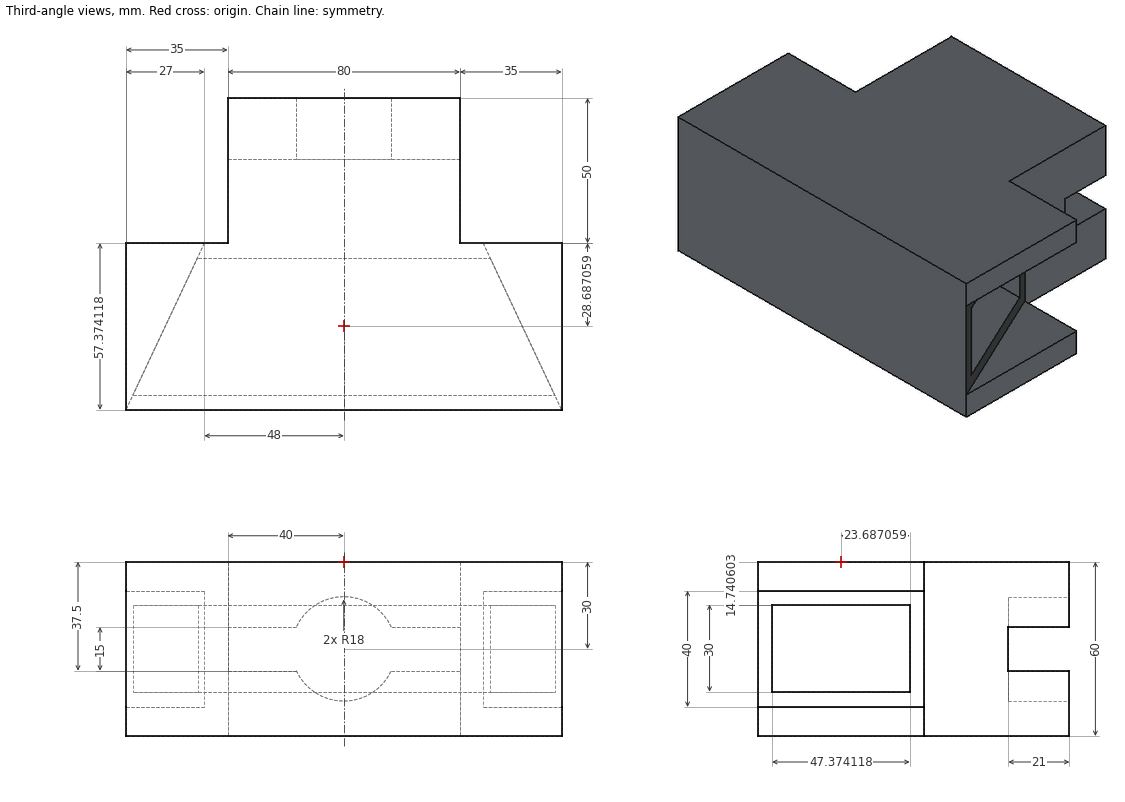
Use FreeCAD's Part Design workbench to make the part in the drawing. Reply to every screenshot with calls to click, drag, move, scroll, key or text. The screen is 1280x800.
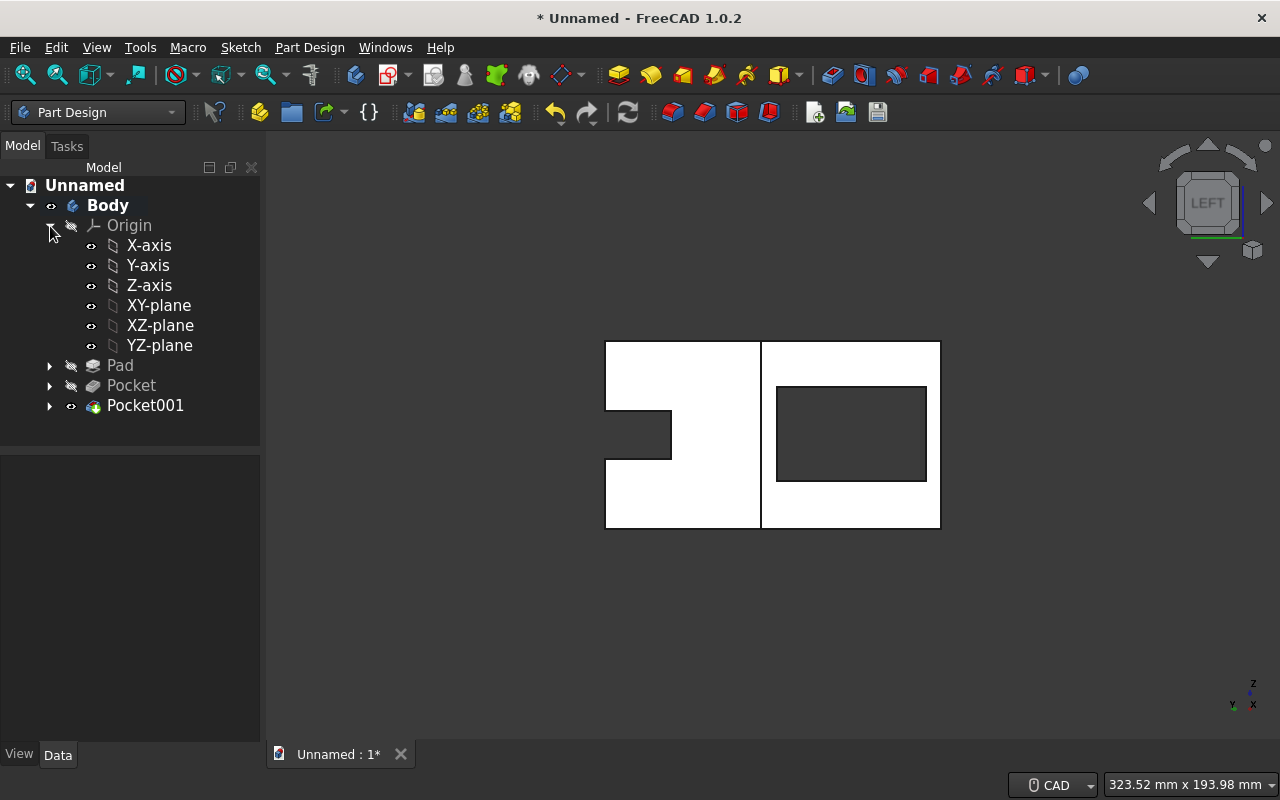
click(136, 306)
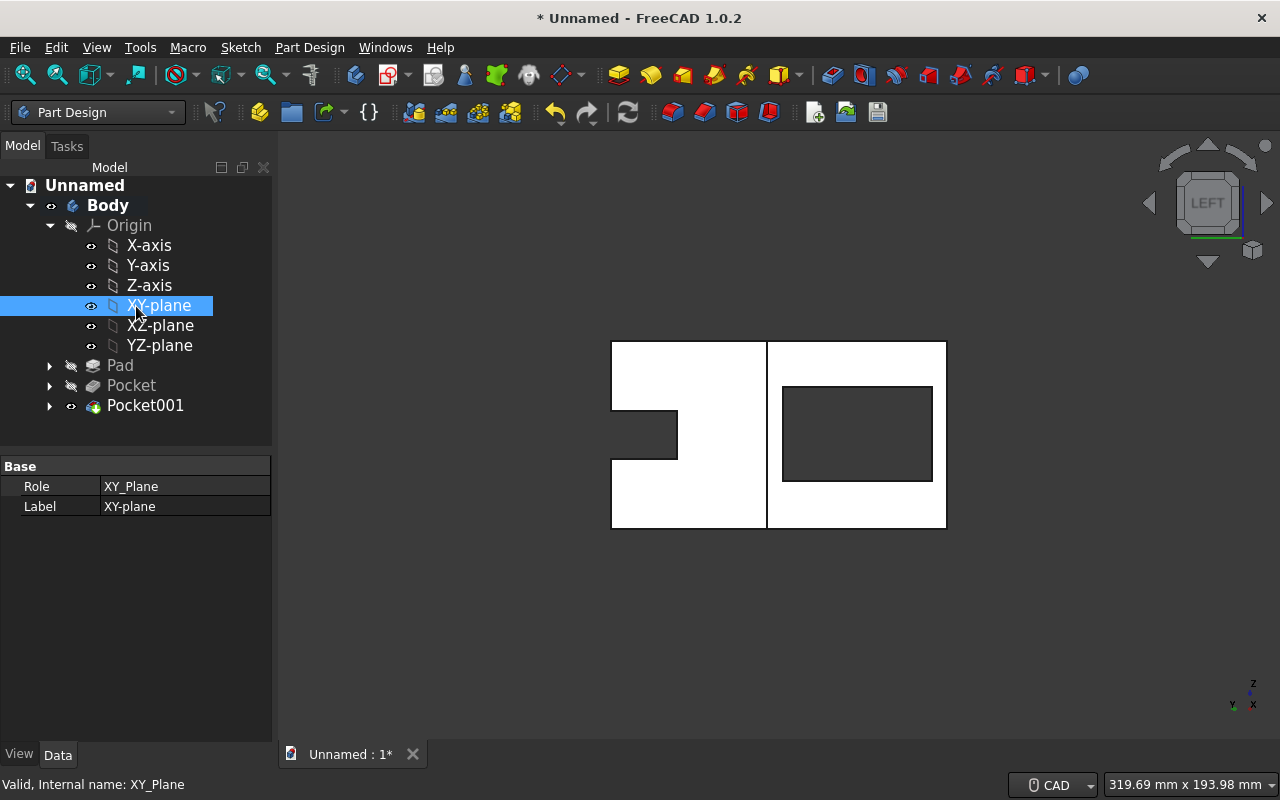
click(562, 76)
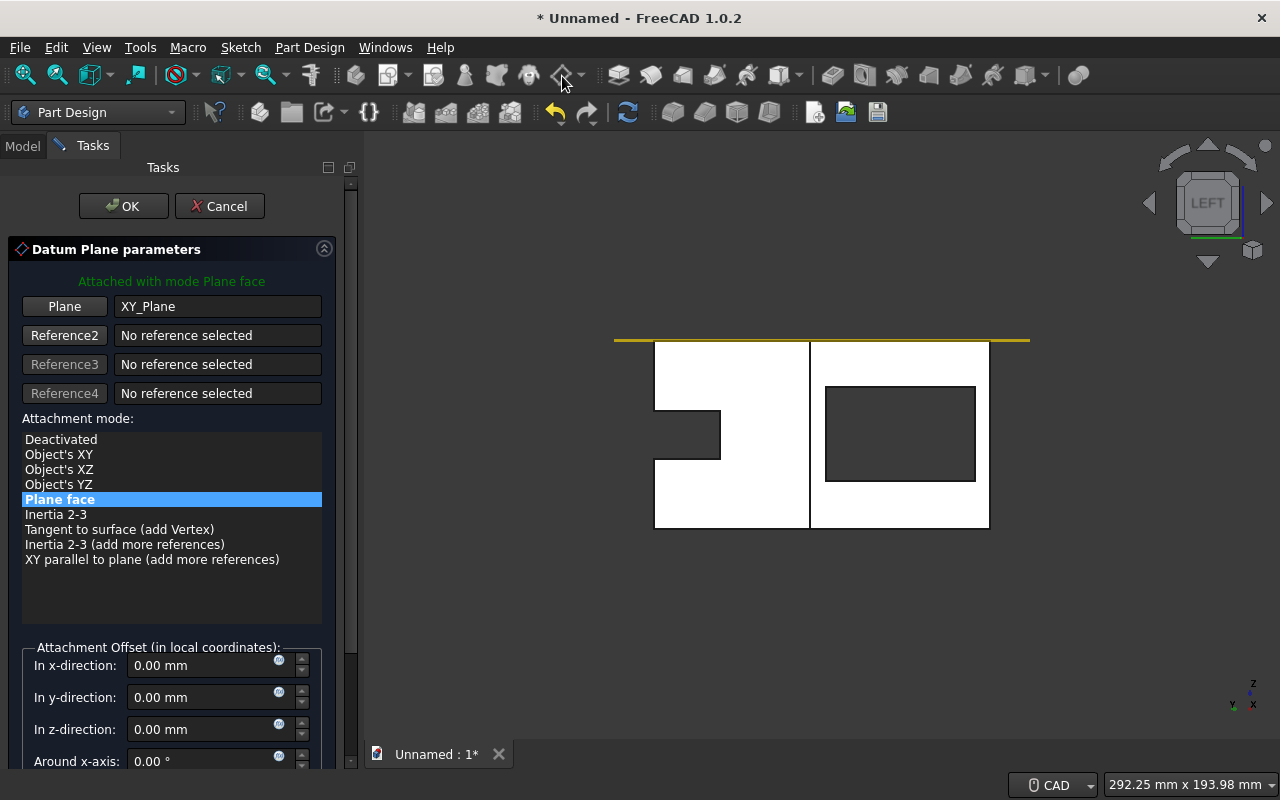
triple_click(210, 729)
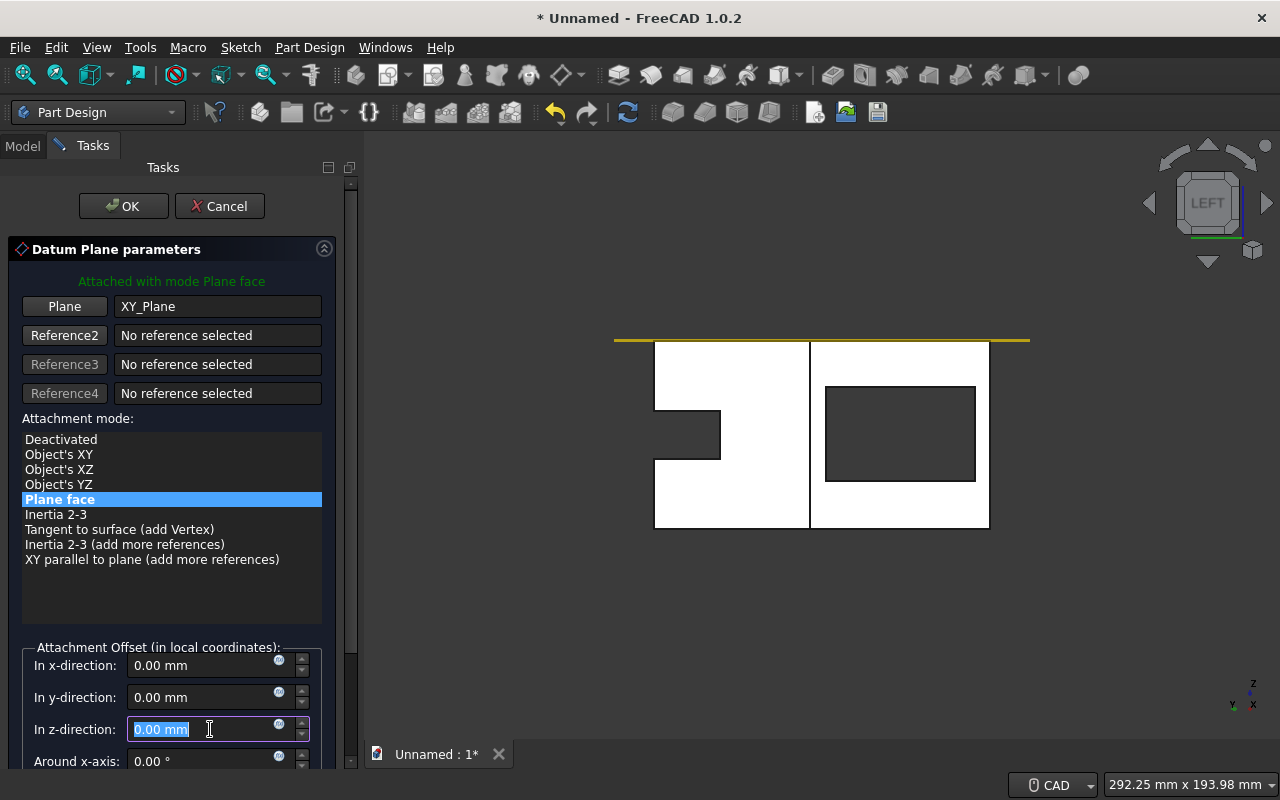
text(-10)
key(Tab)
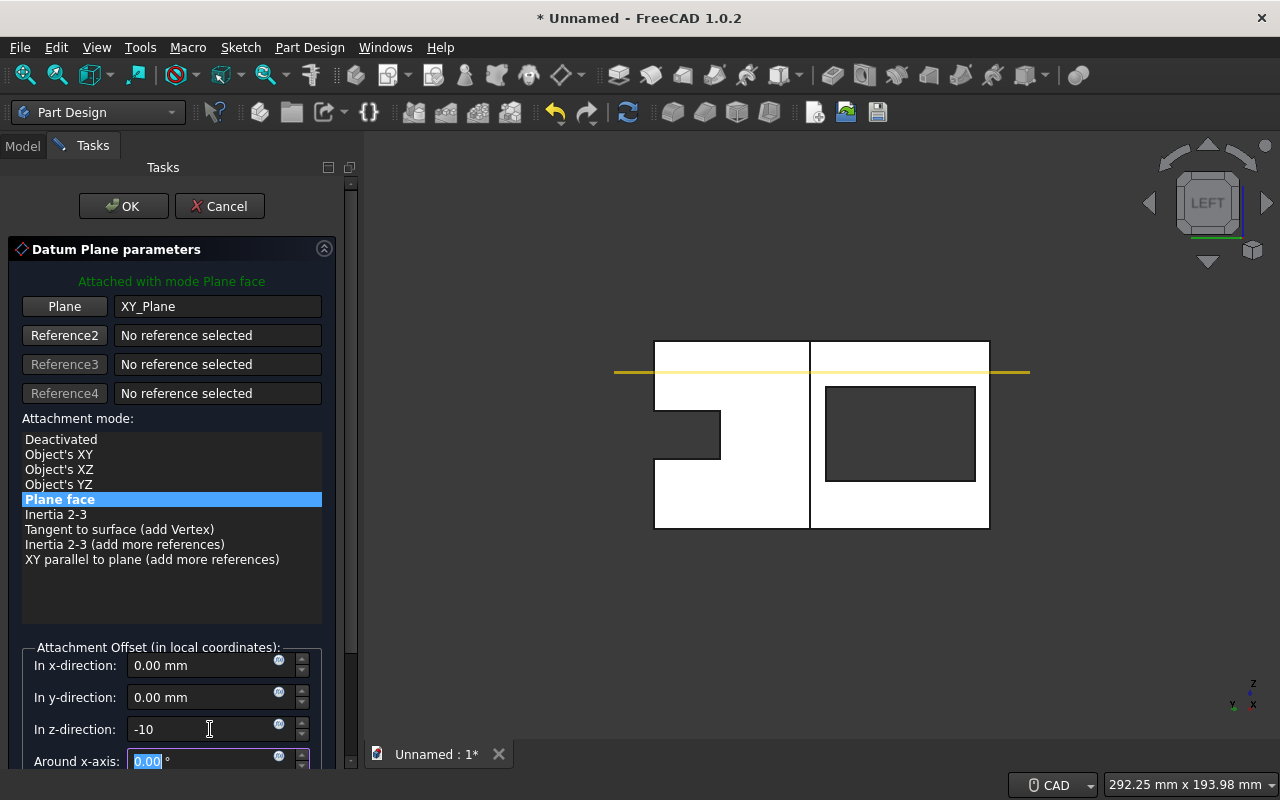
click(124, 206)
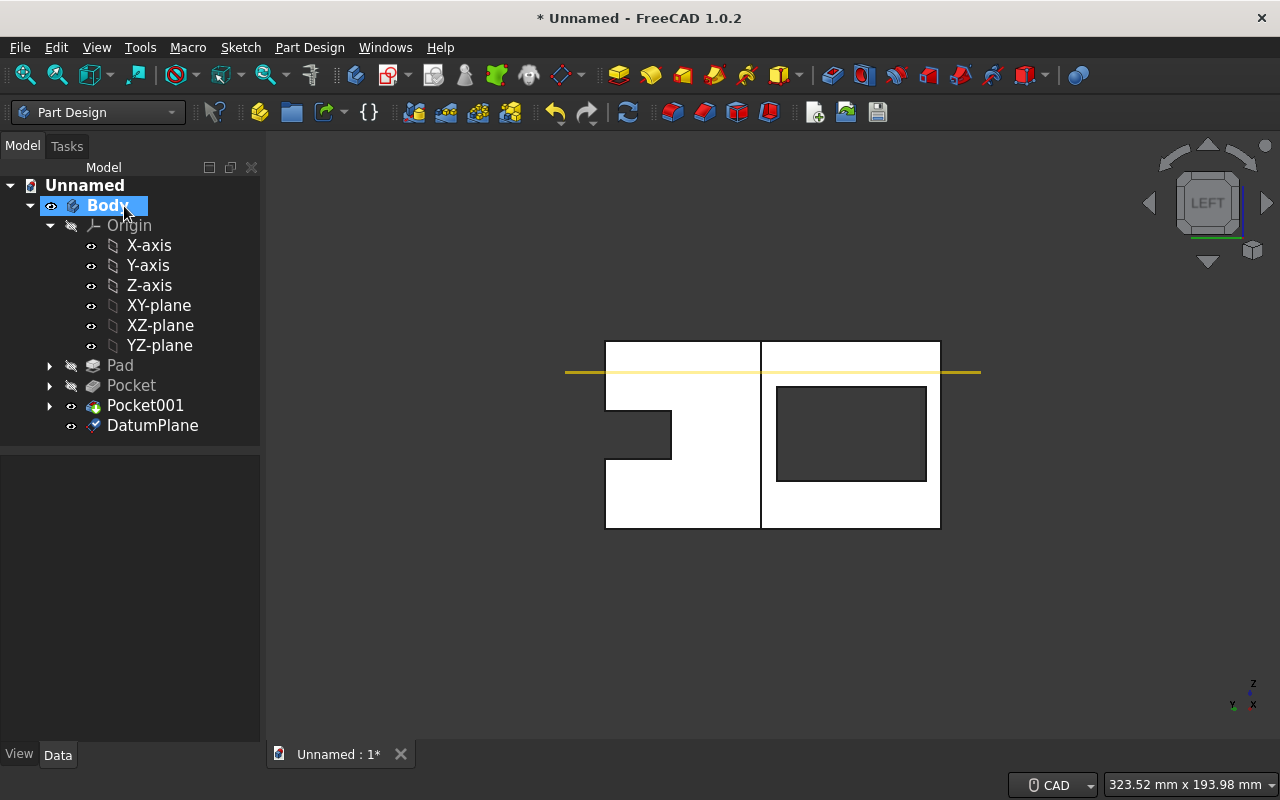
click(116, 426)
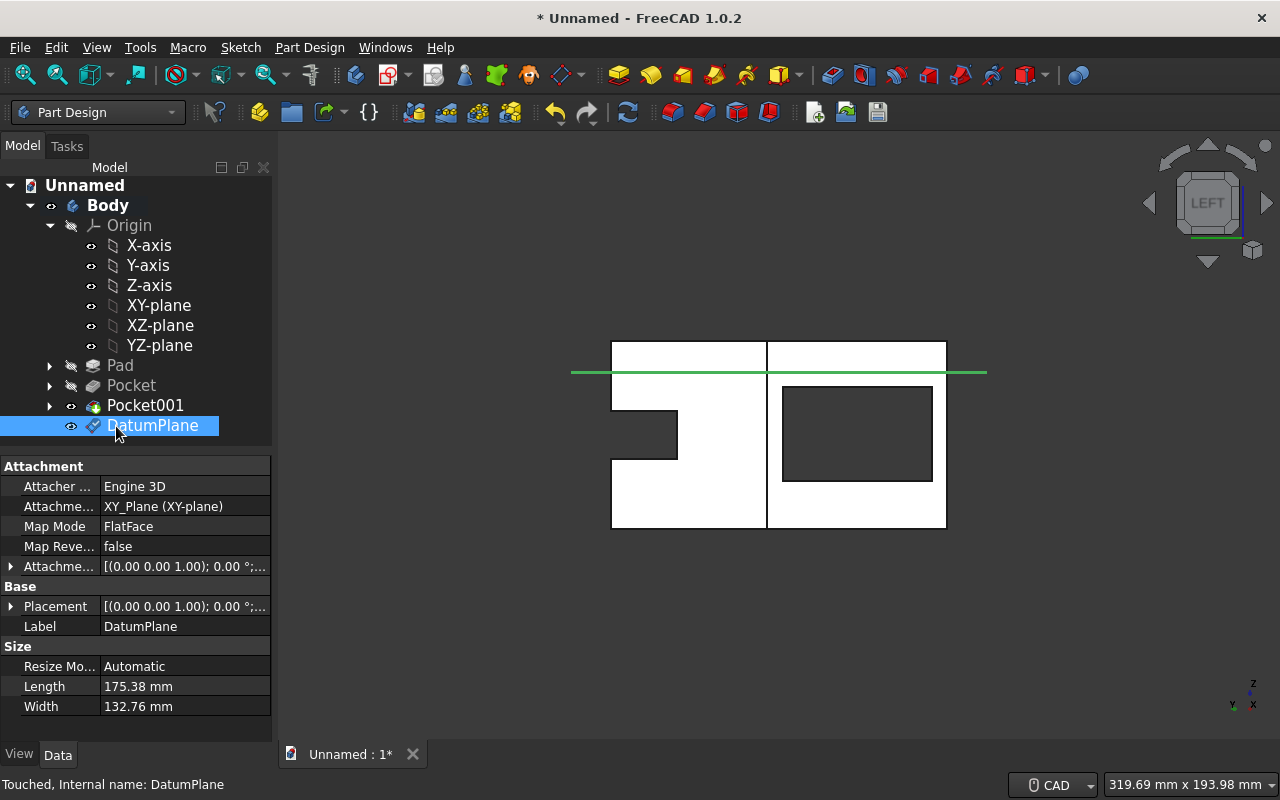
click(388, 76)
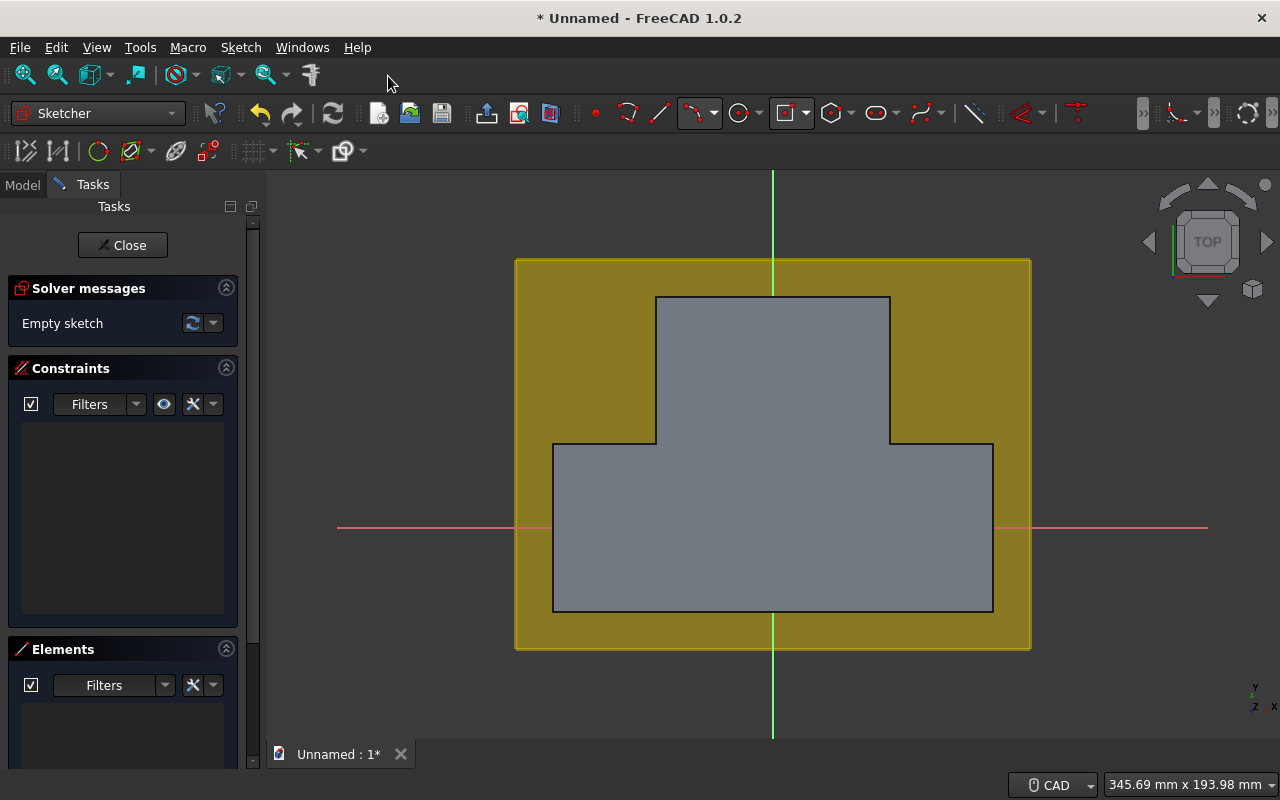
click(552, 114)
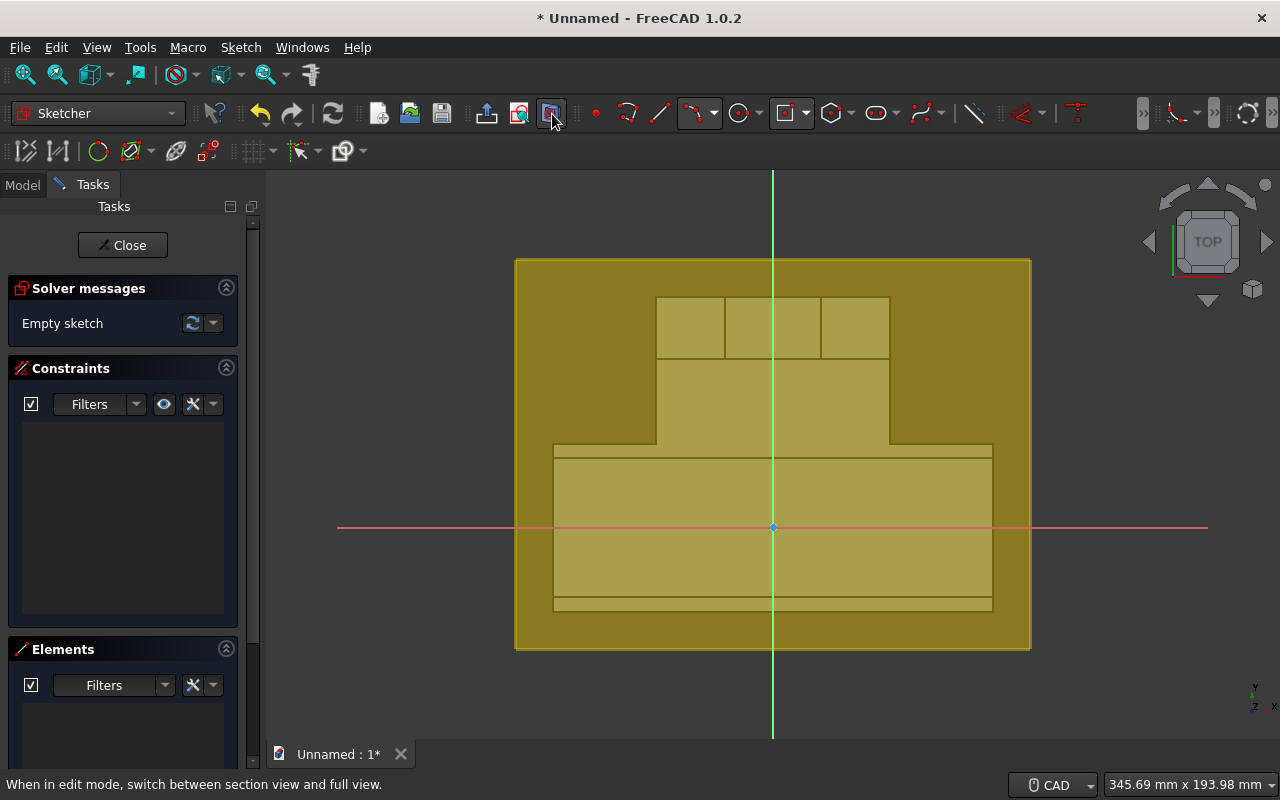
key(g)
key(m)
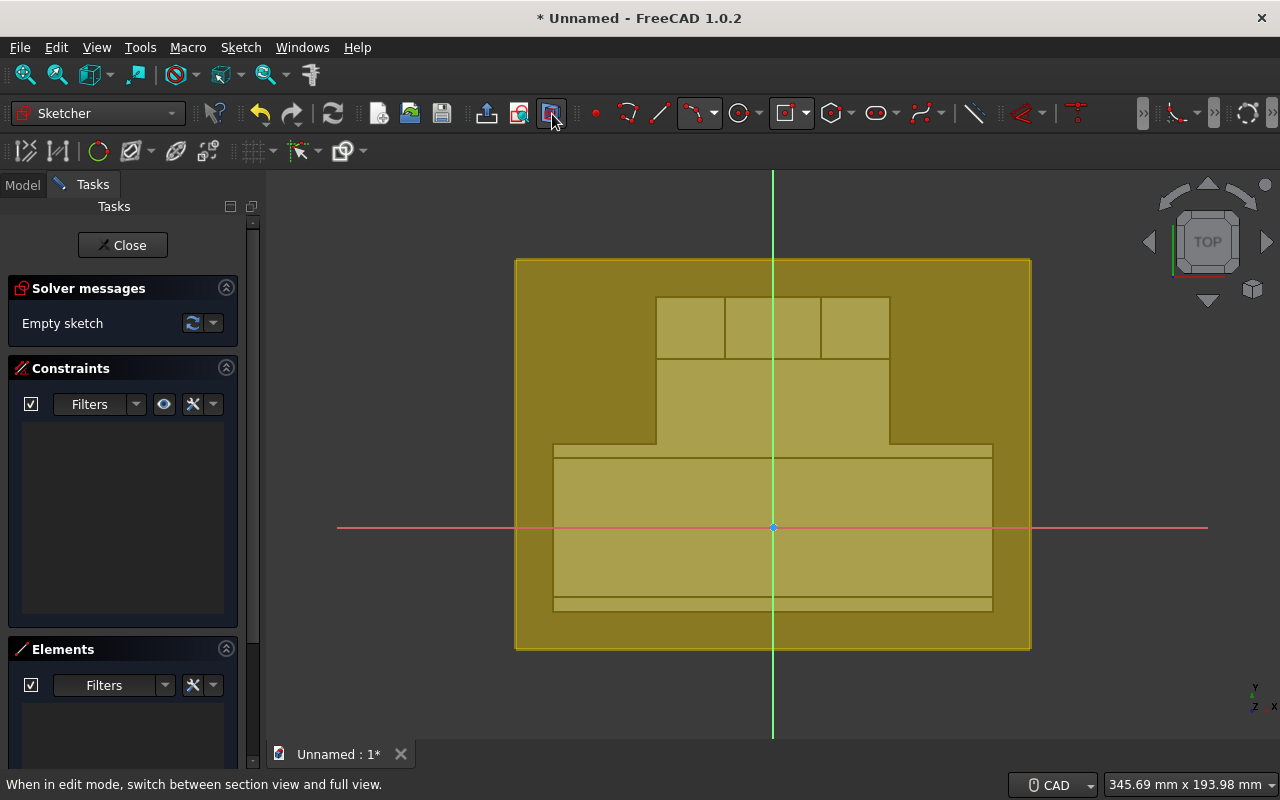
click(632, 444)
click(553, 444)
click(553, 612)
click(632, 445)